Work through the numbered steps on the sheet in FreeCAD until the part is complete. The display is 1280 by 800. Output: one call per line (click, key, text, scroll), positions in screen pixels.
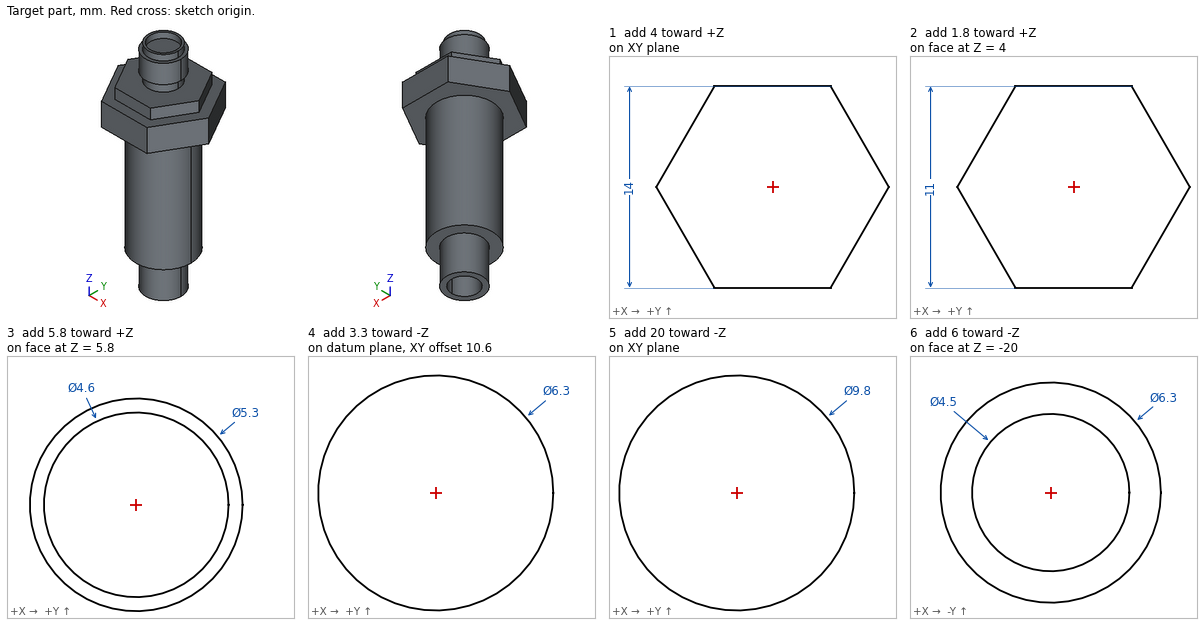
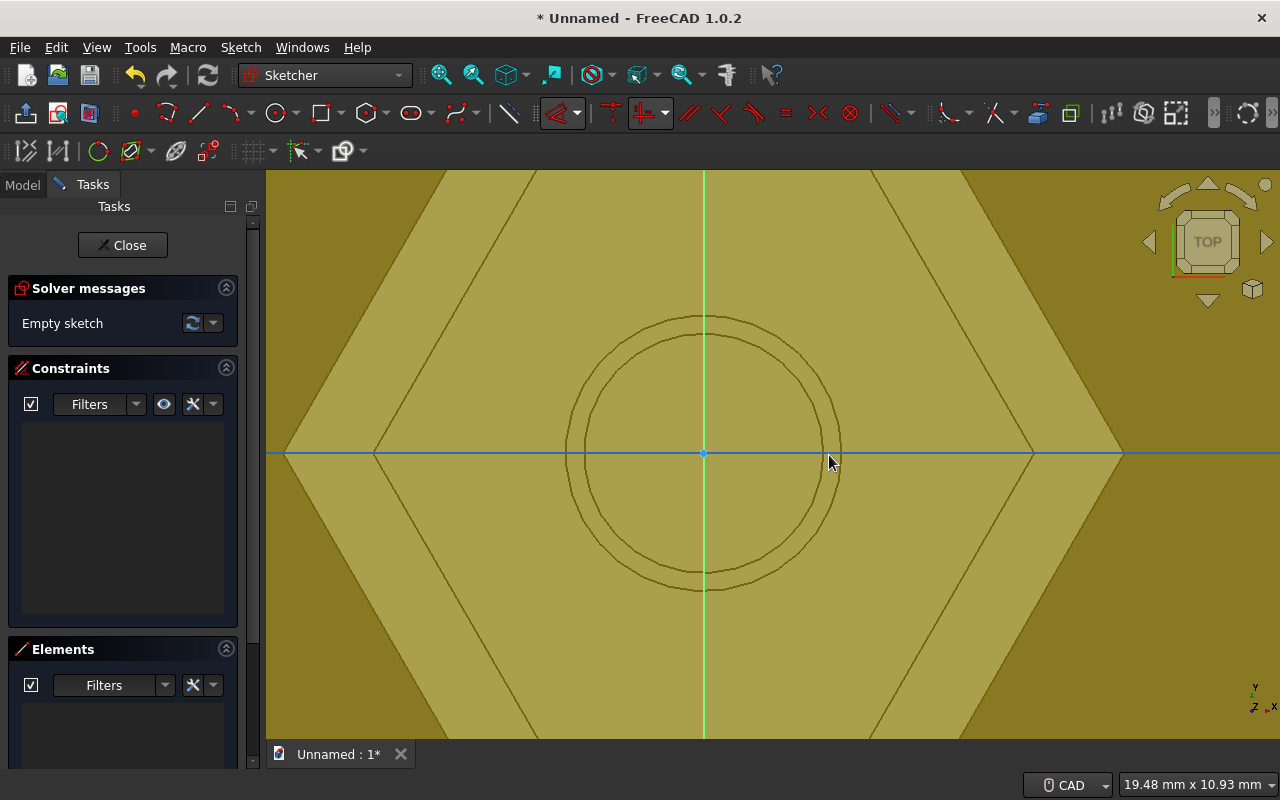
click(276, 114)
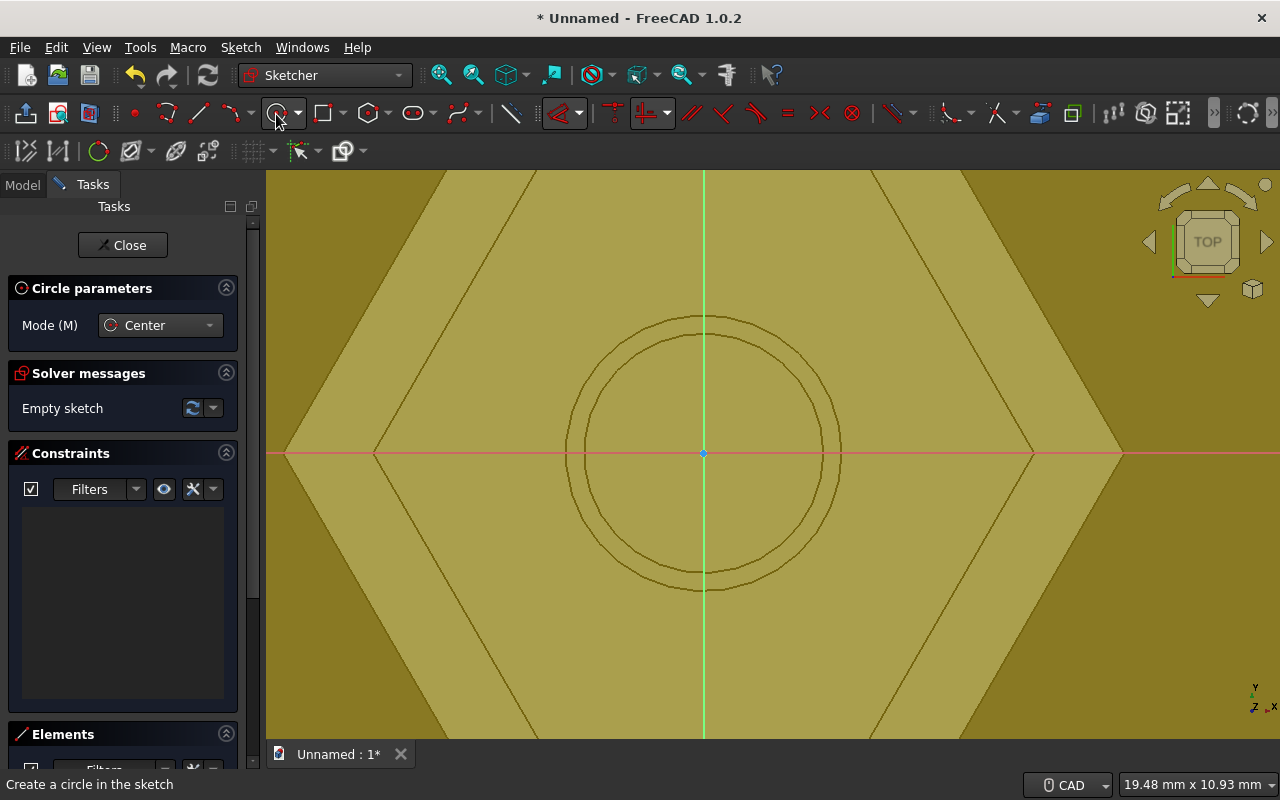
click(704, 453)
click(820, 337)
key(Escape)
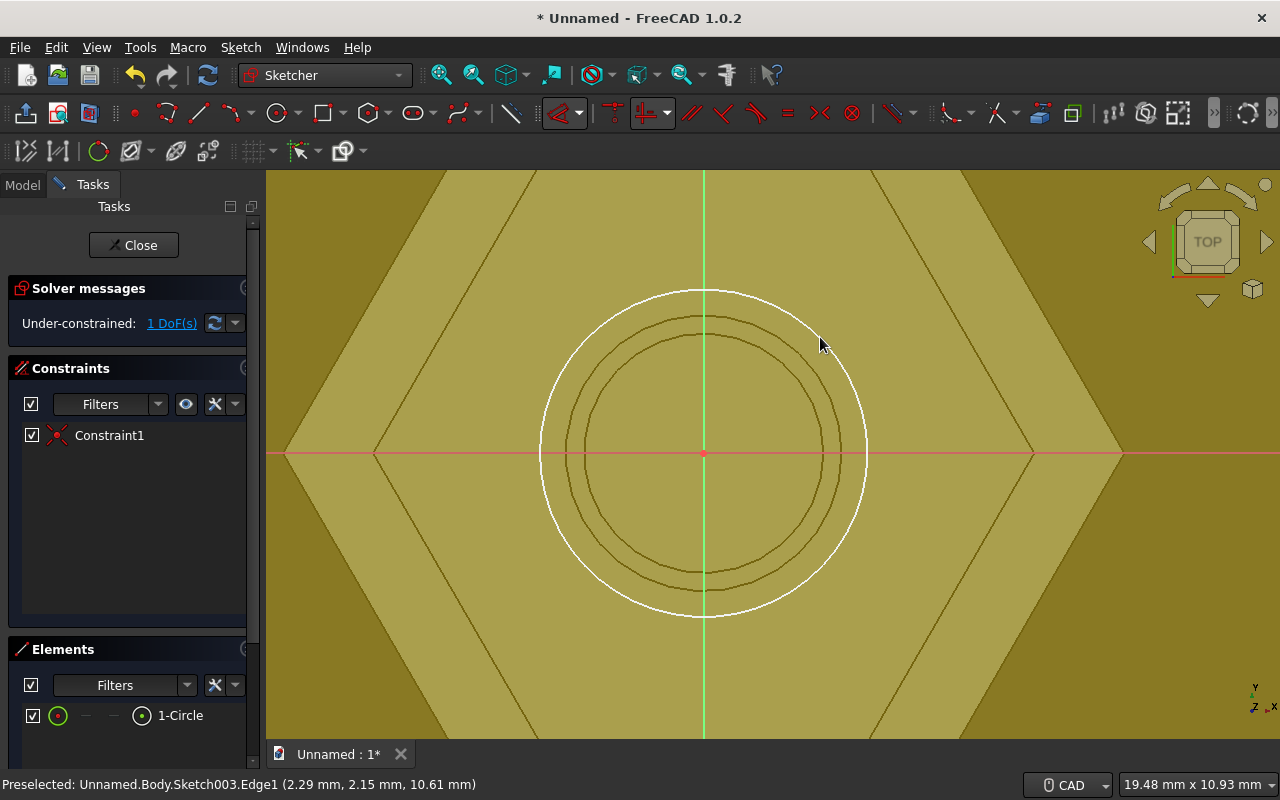
click(819, 337)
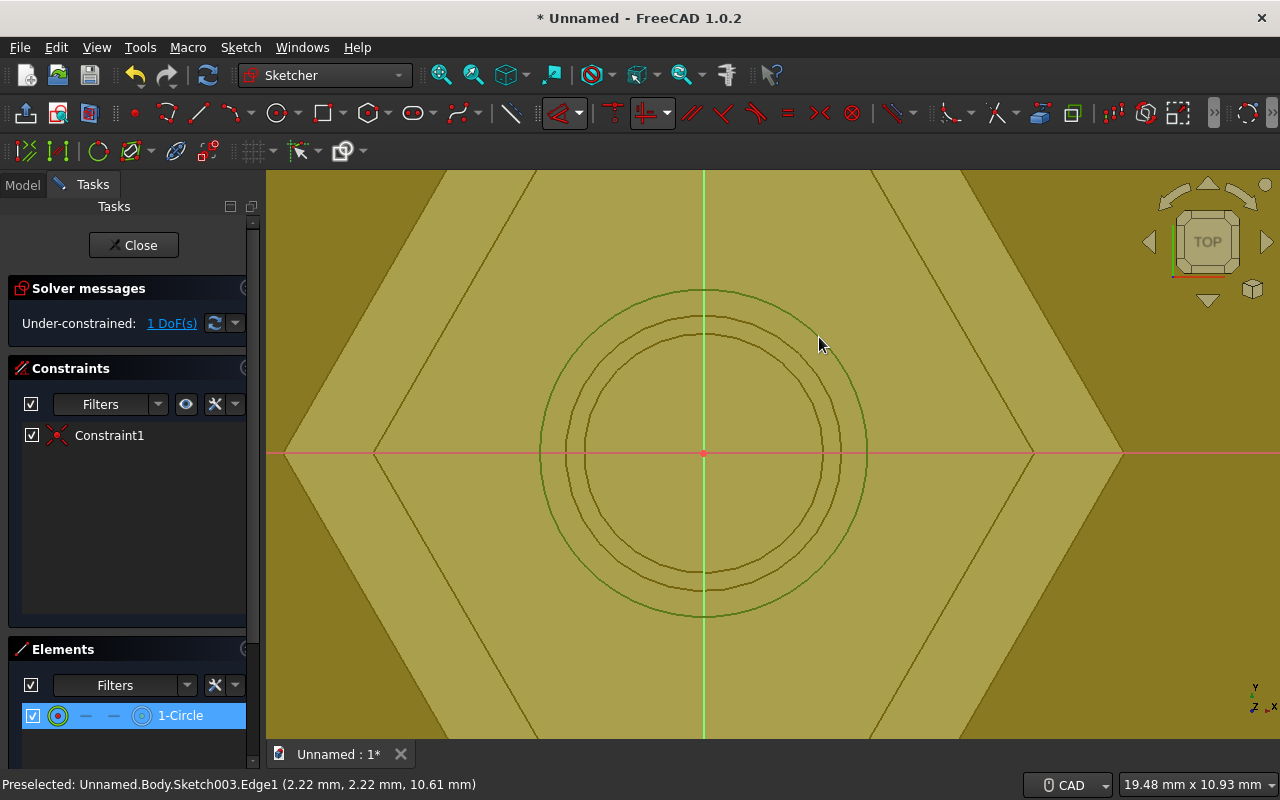
click(582, 114)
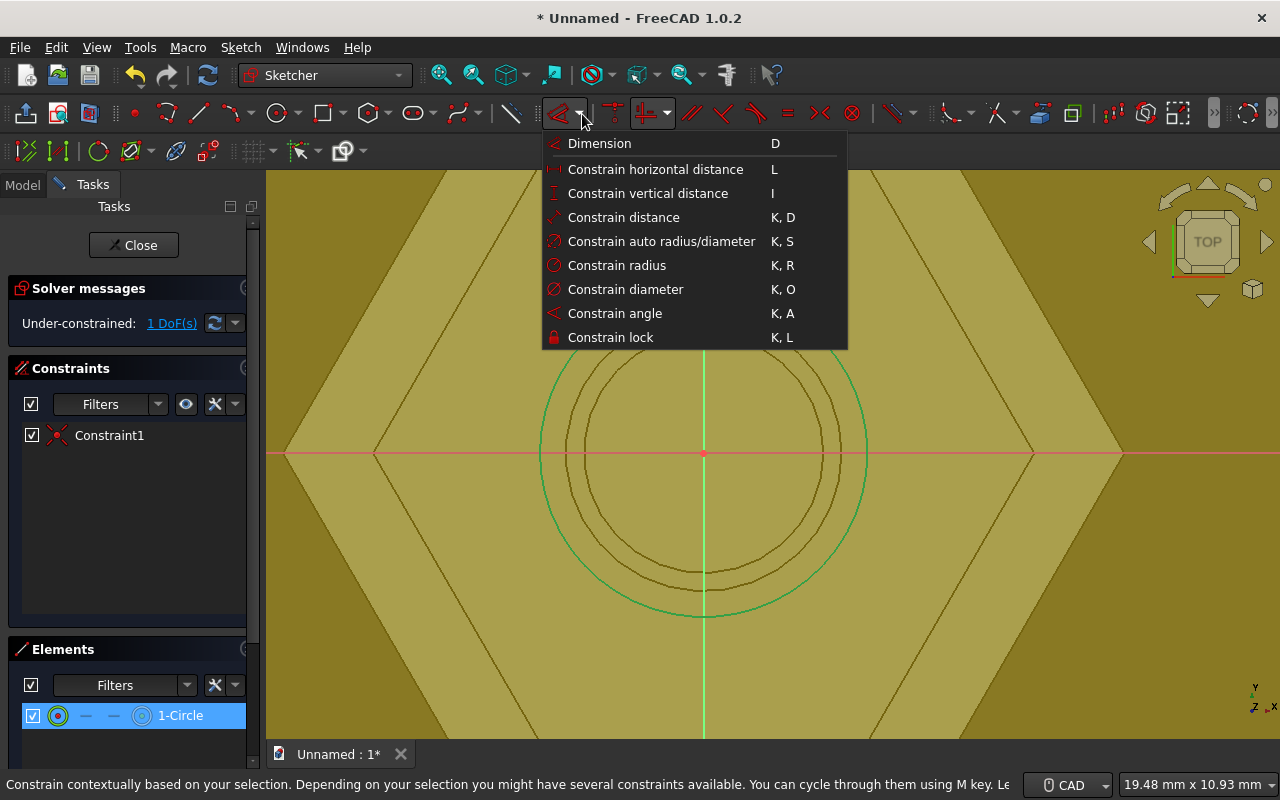
click(695, 289)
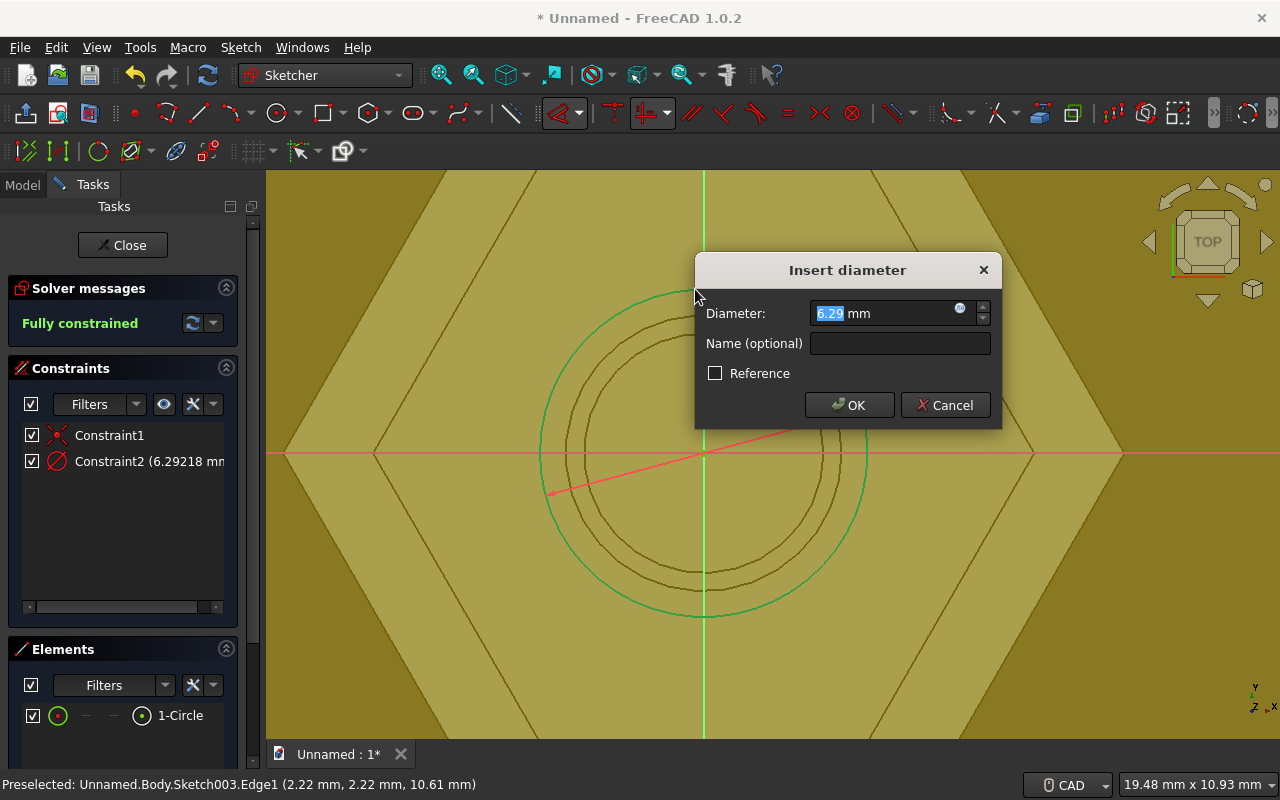
text(6.3)
key(Return)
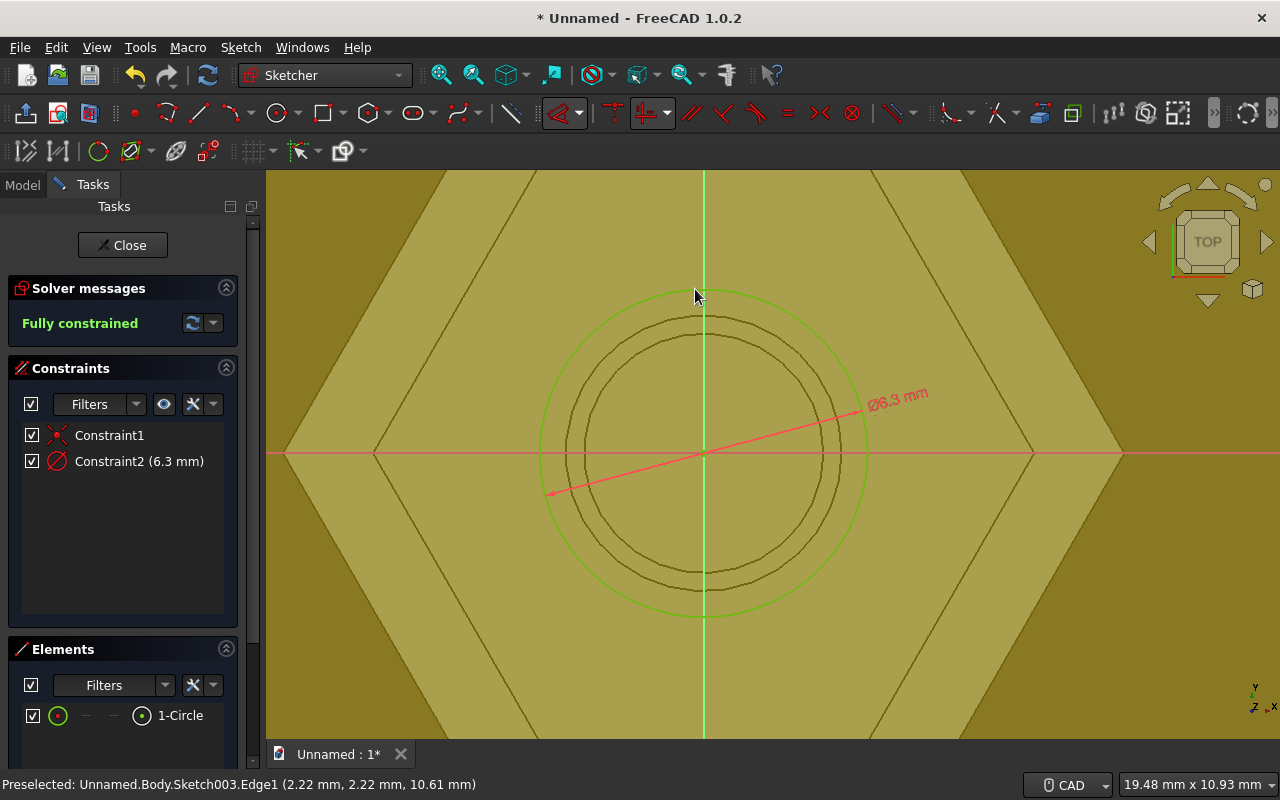
click(123, 245)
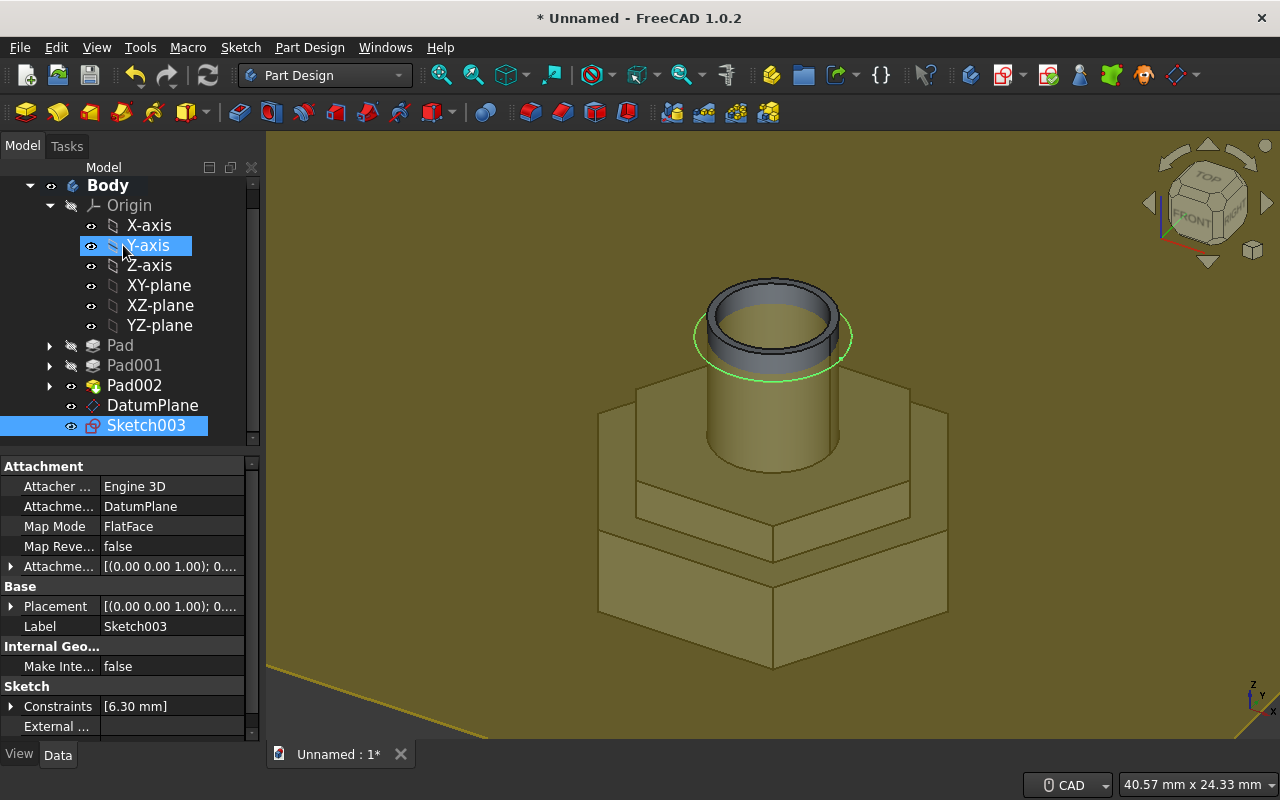
click(26, 112)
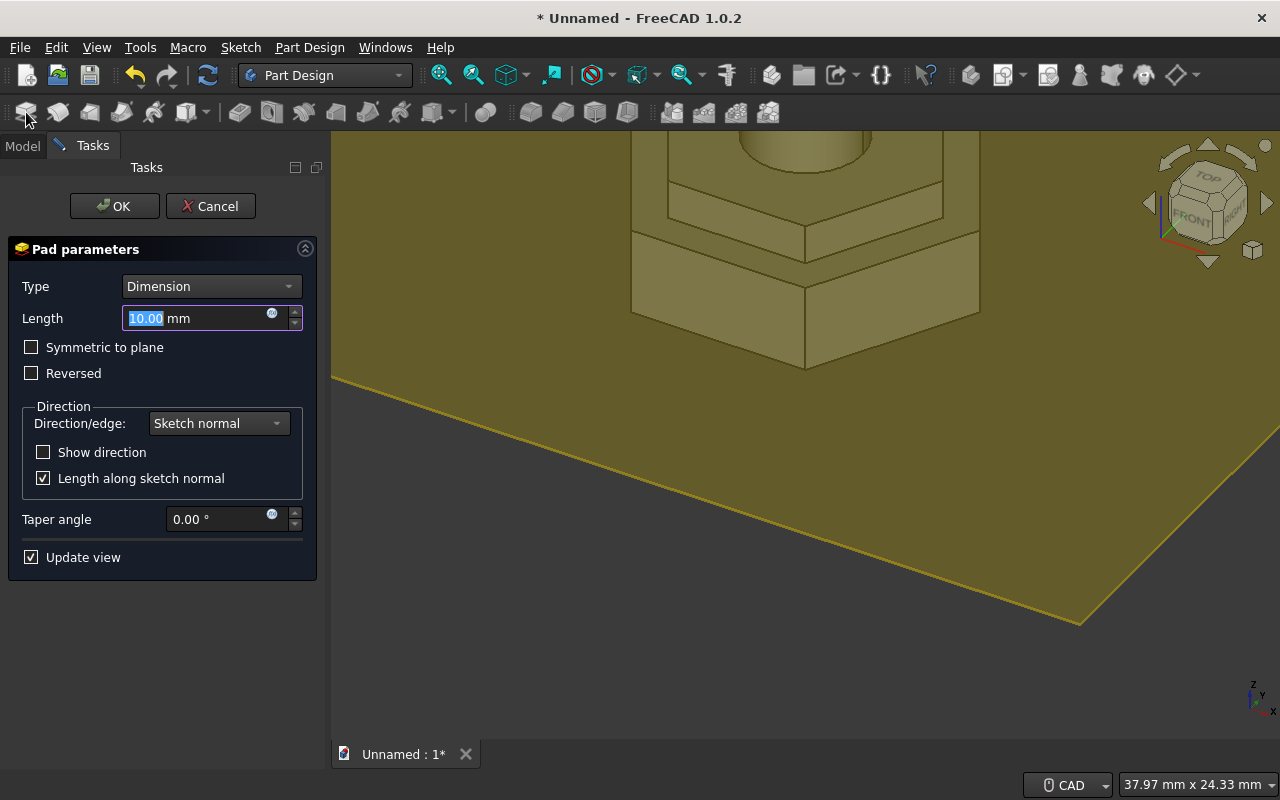
text(3.3)
key(Tab)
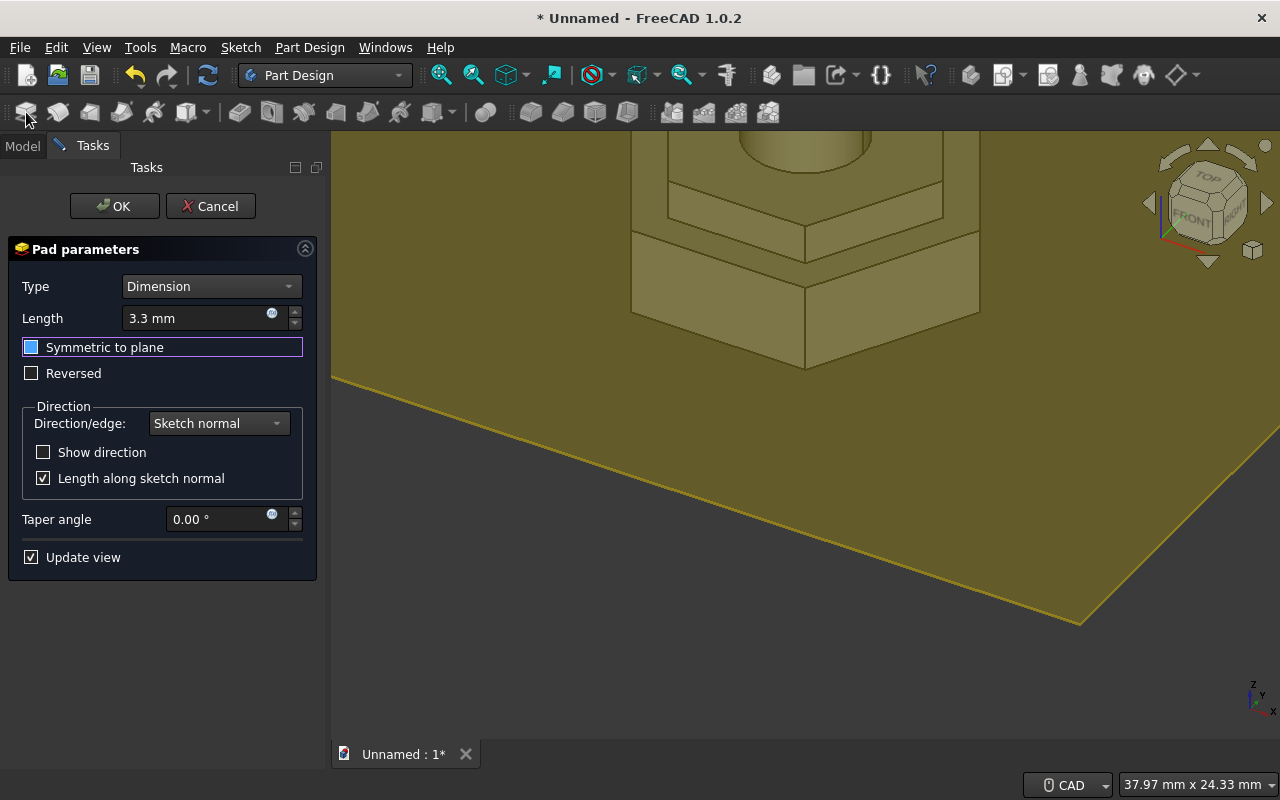
click(30, 373)